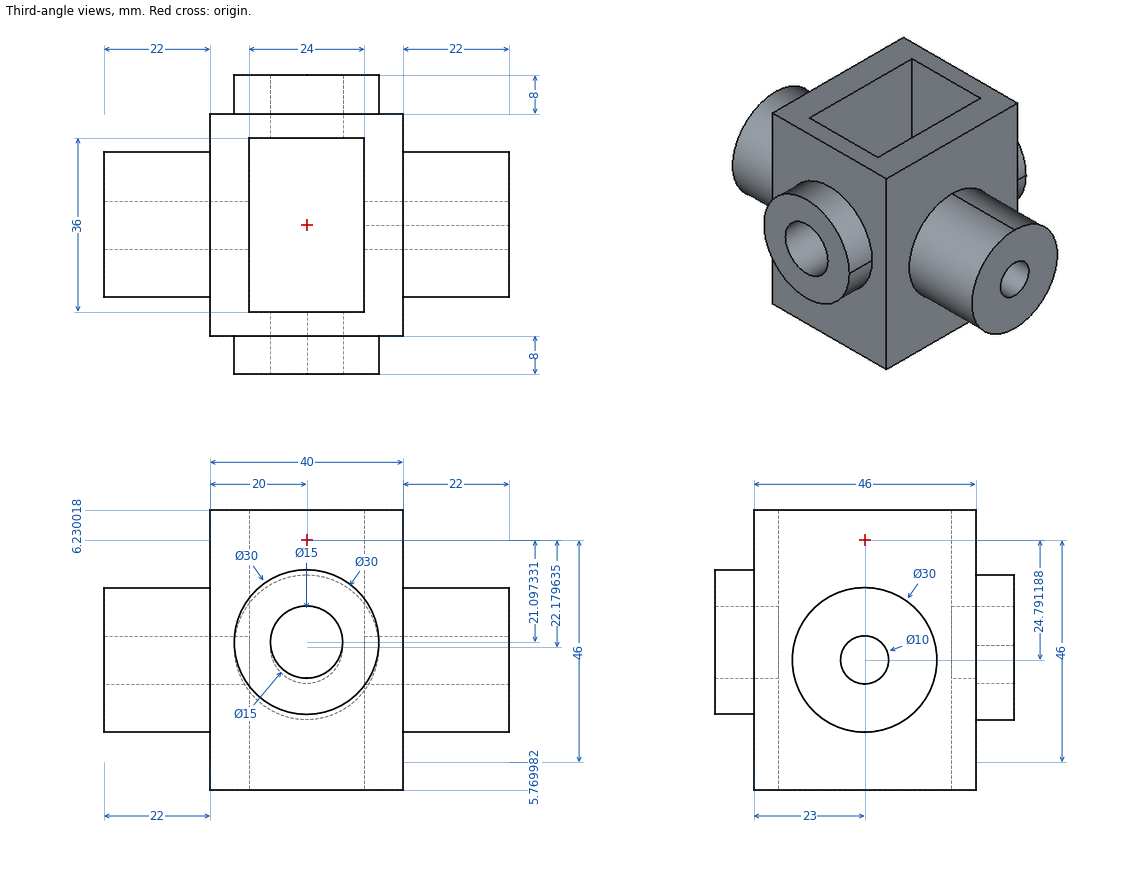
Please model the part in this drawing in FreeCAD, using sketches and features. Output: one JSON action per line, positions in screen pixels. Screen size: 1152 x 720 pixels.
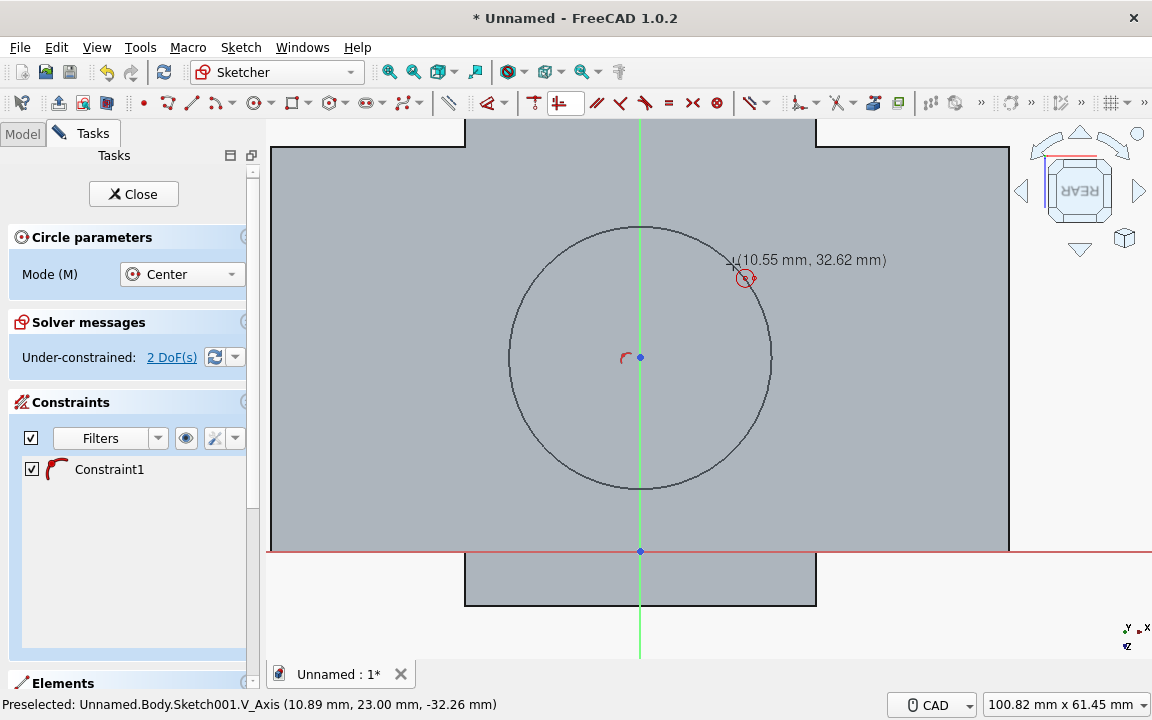
{"action": "left_click", "coordinate": [640, 358]}
{"action": "left_click", "coordinate": [687, 310]}
{"action": "key", "text": "Escape"}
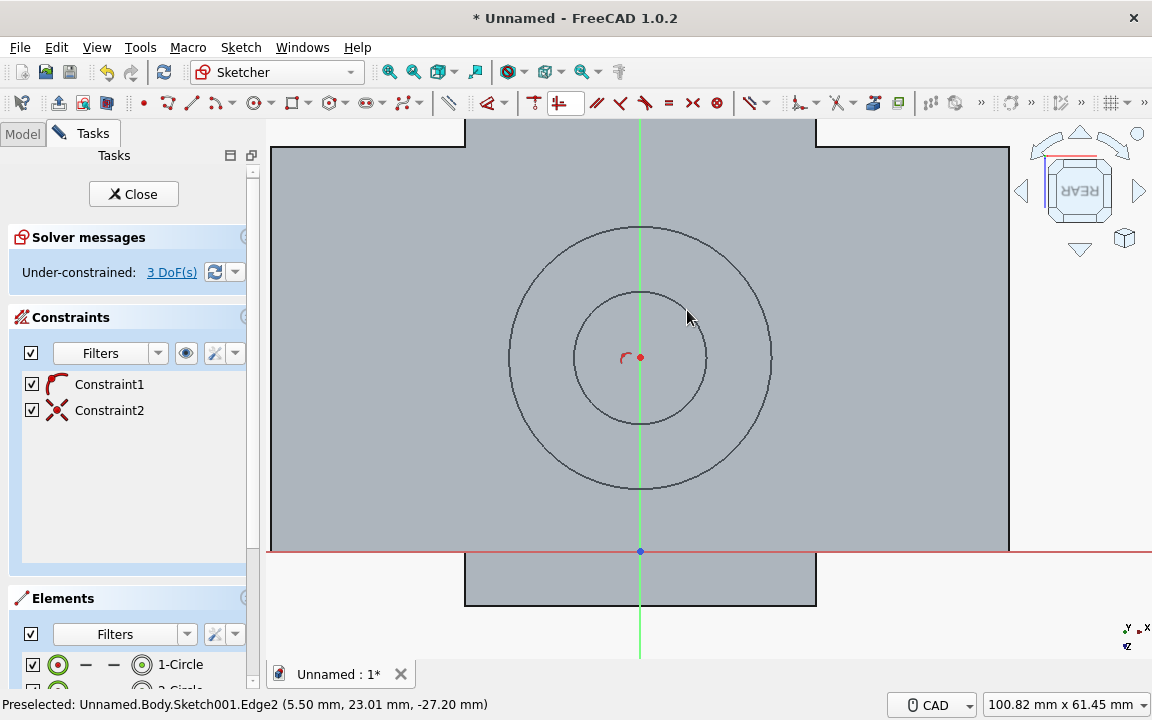
{"action": "key", "text": "d"}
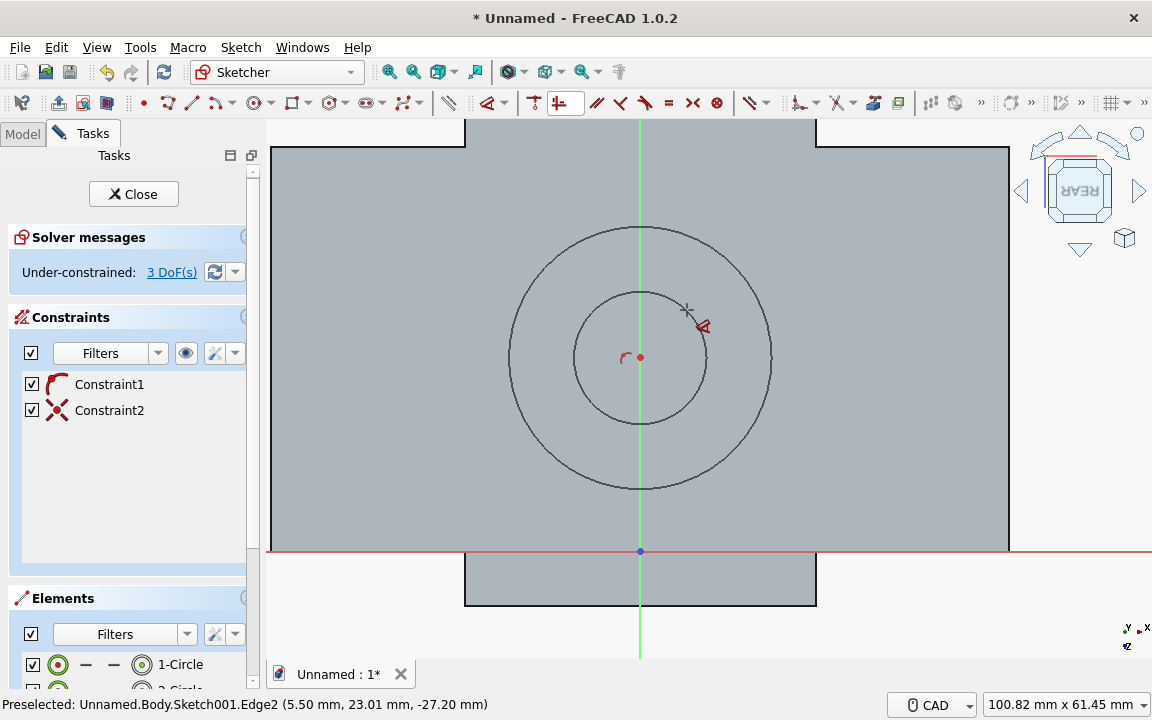
{"action": "left_click", "coordinate": [733, 265]}
{"action": "left_click", "coordinate": [756, 242]}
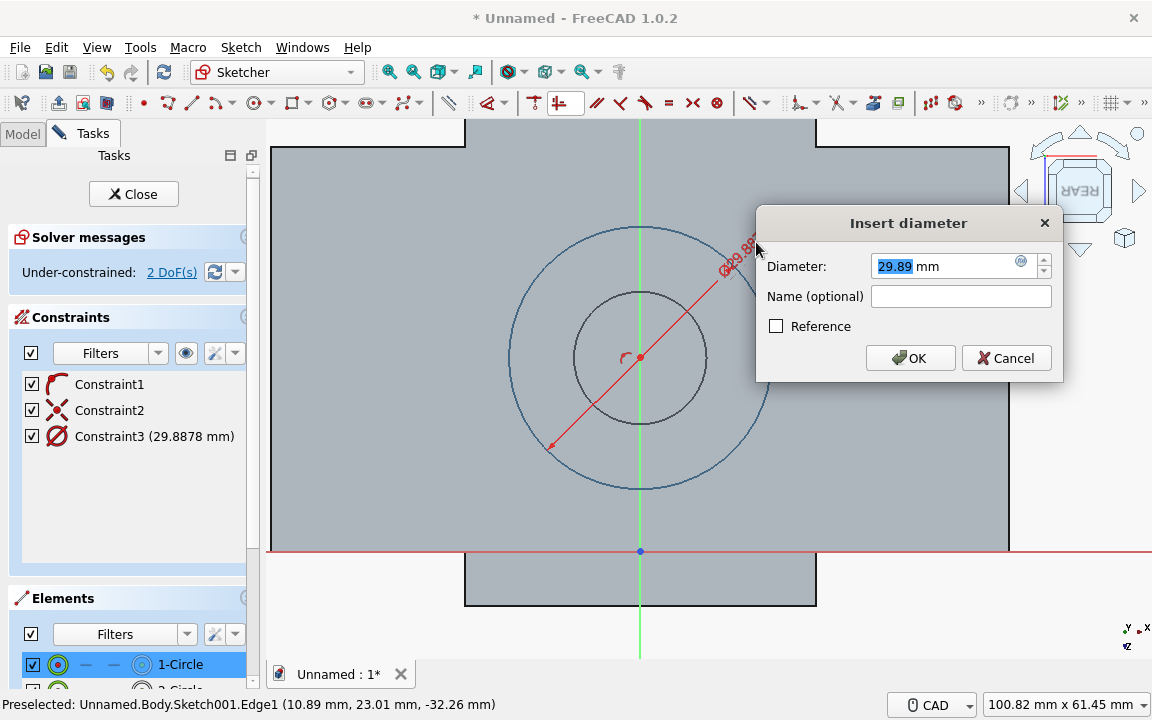
{"action": "type", "text": "30"}
{"action": "key", "text": "Return"}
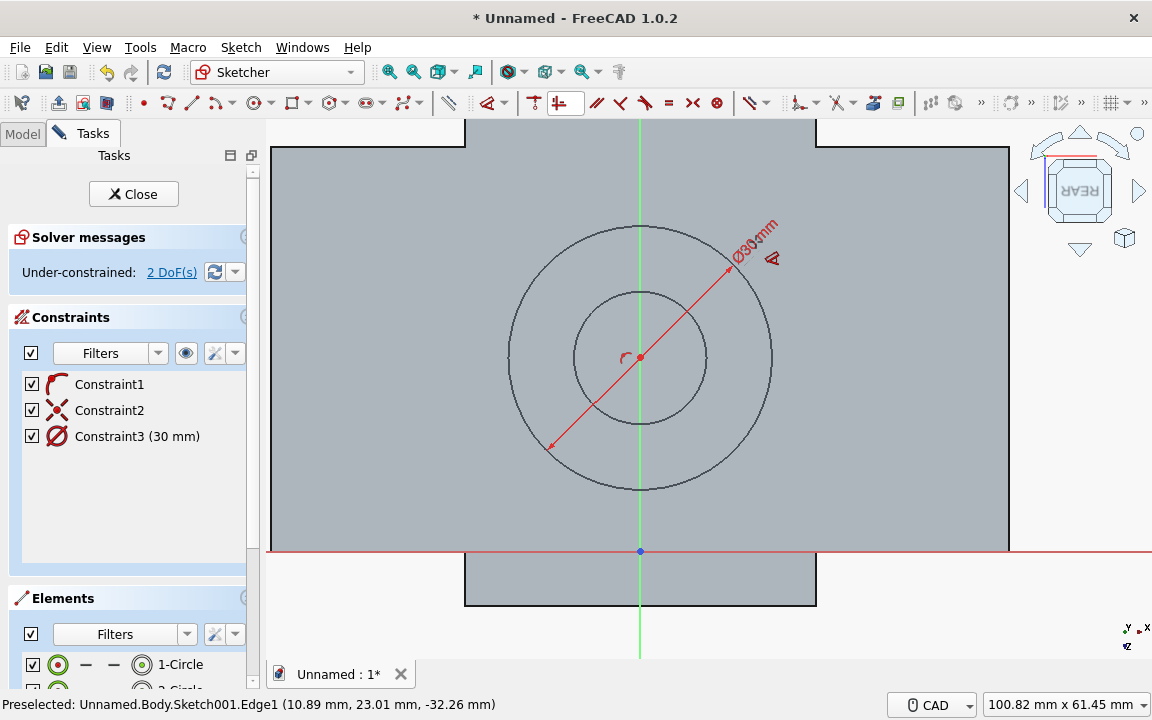
{"action": "left_click", "coordinate": [687, 311]}
{"action": "left_click", "coordinate": [710, 288]}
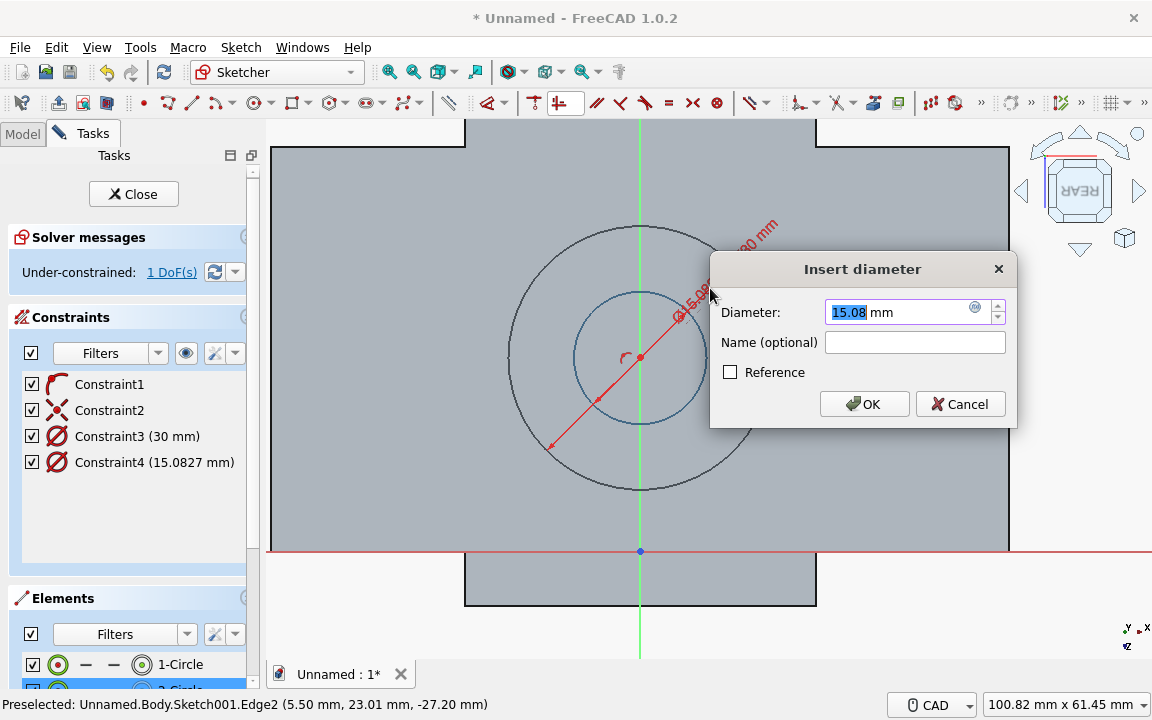
{"action": "type", "text": "15"}
{"action": "key", "text": "Return"}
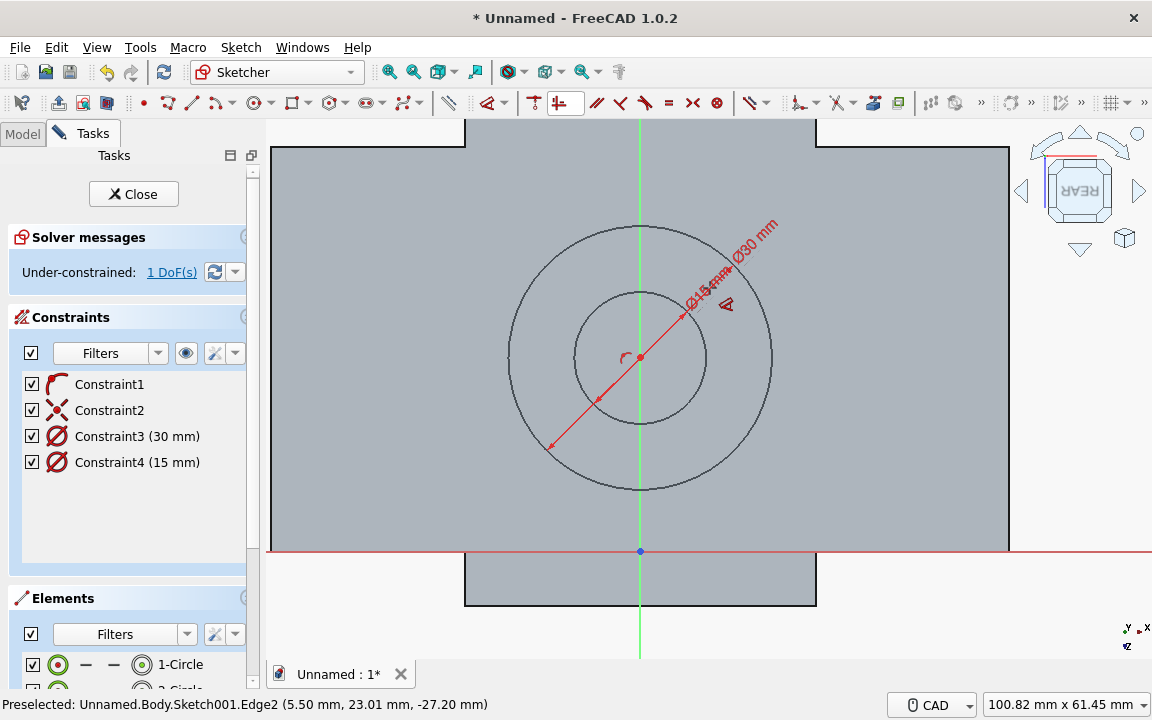
{"action": "left_click", "coordinate": [640, 358]}
{"action": "left_click", "coordinate": [674, 455]}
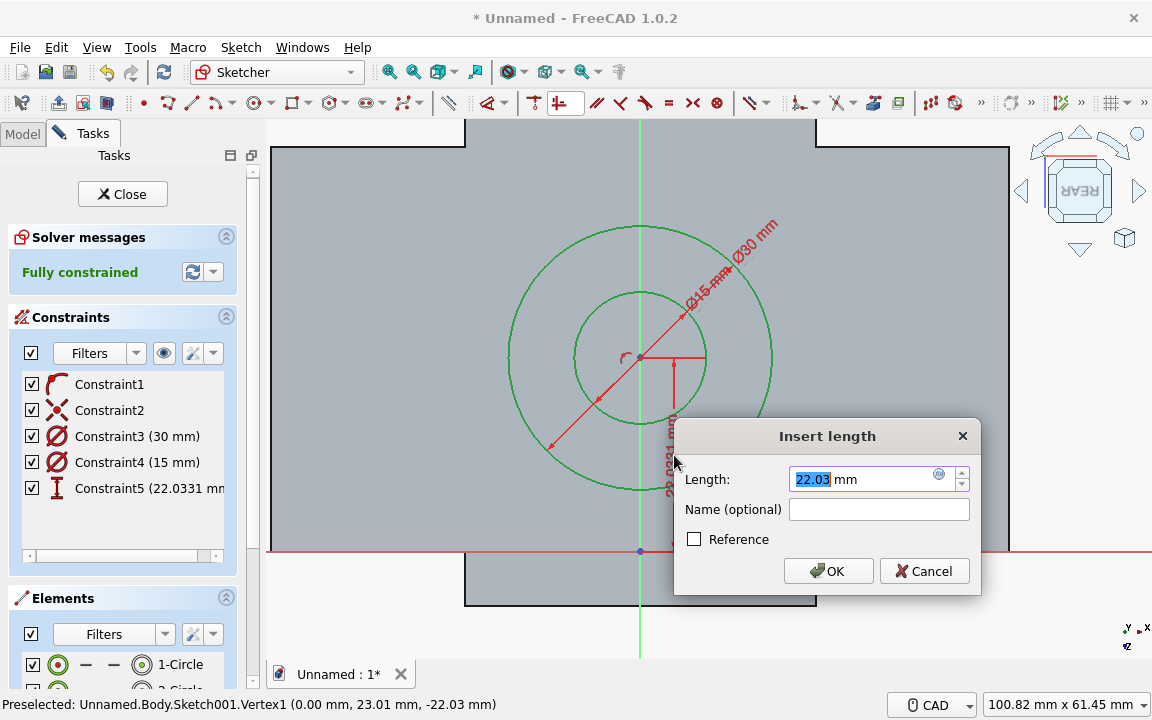
{"action": "type", "text": "22.179635"}
{"action": "key", "text": "Return"}
{"action": "key", "text": "Escape"}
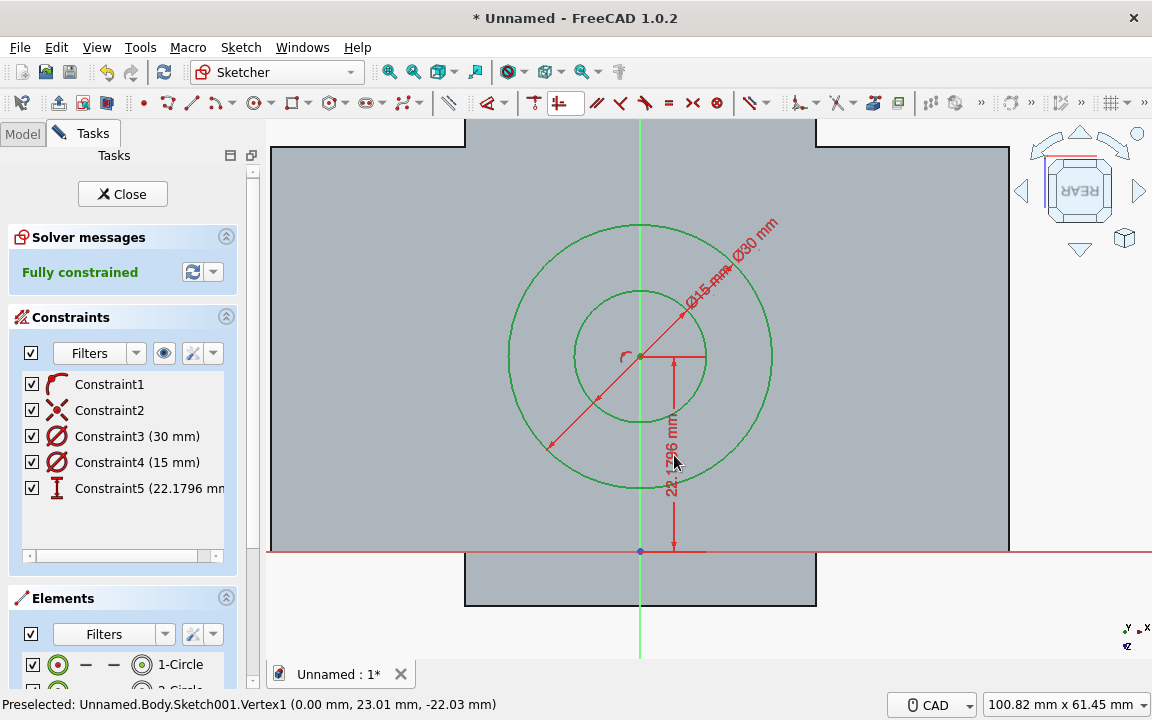
{"action": "left_click", "coordinate": [123, 194]}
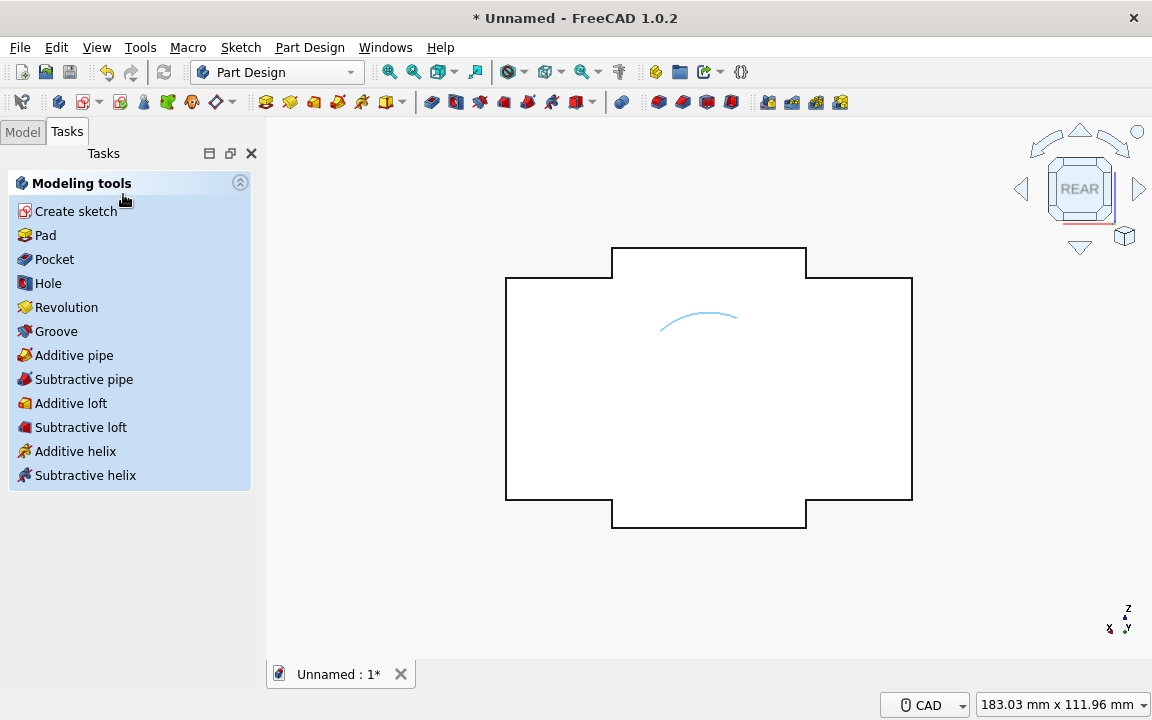
{"action": "left_click", "coordinate": [266, 102]}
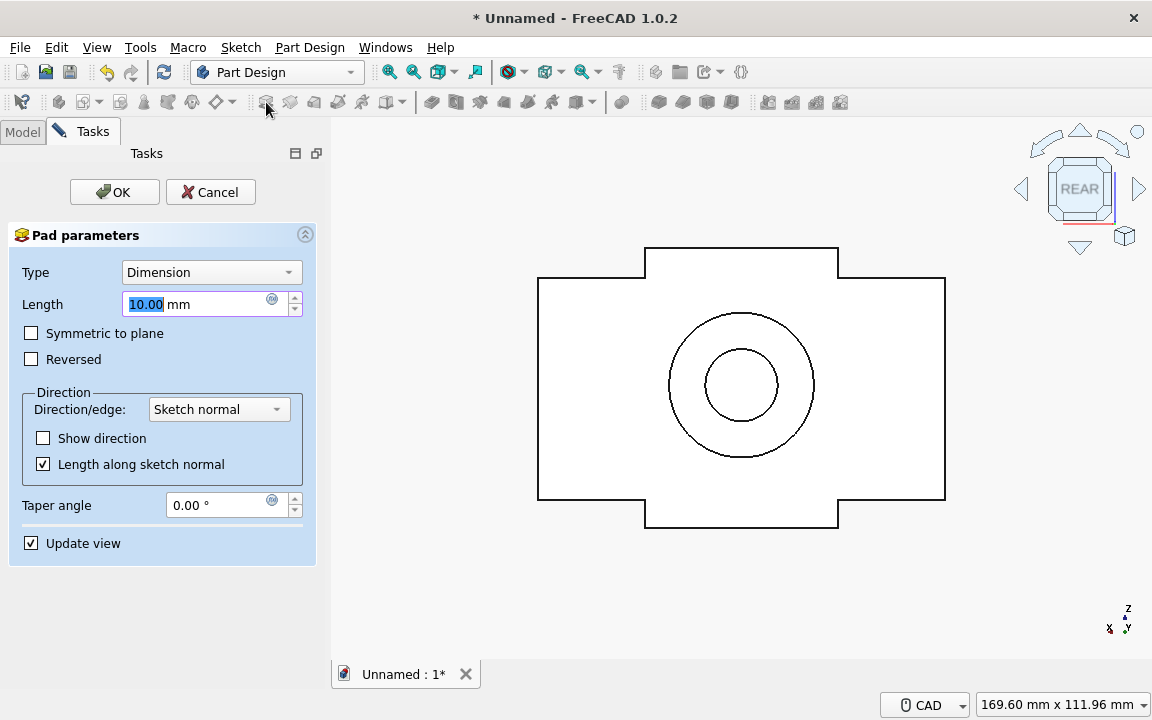
{"action": "type", "text": "8"}
{"action": "key", "text": "Tab"}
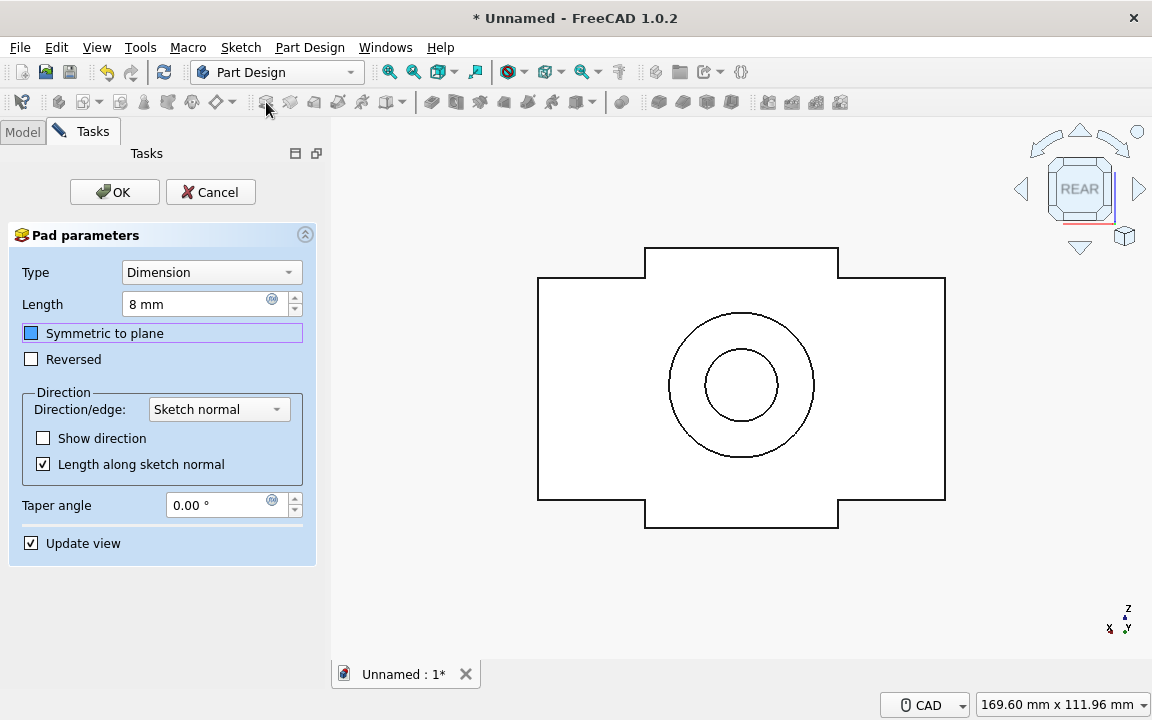
{"action": "left_click", "coordinate": [115, 192]}